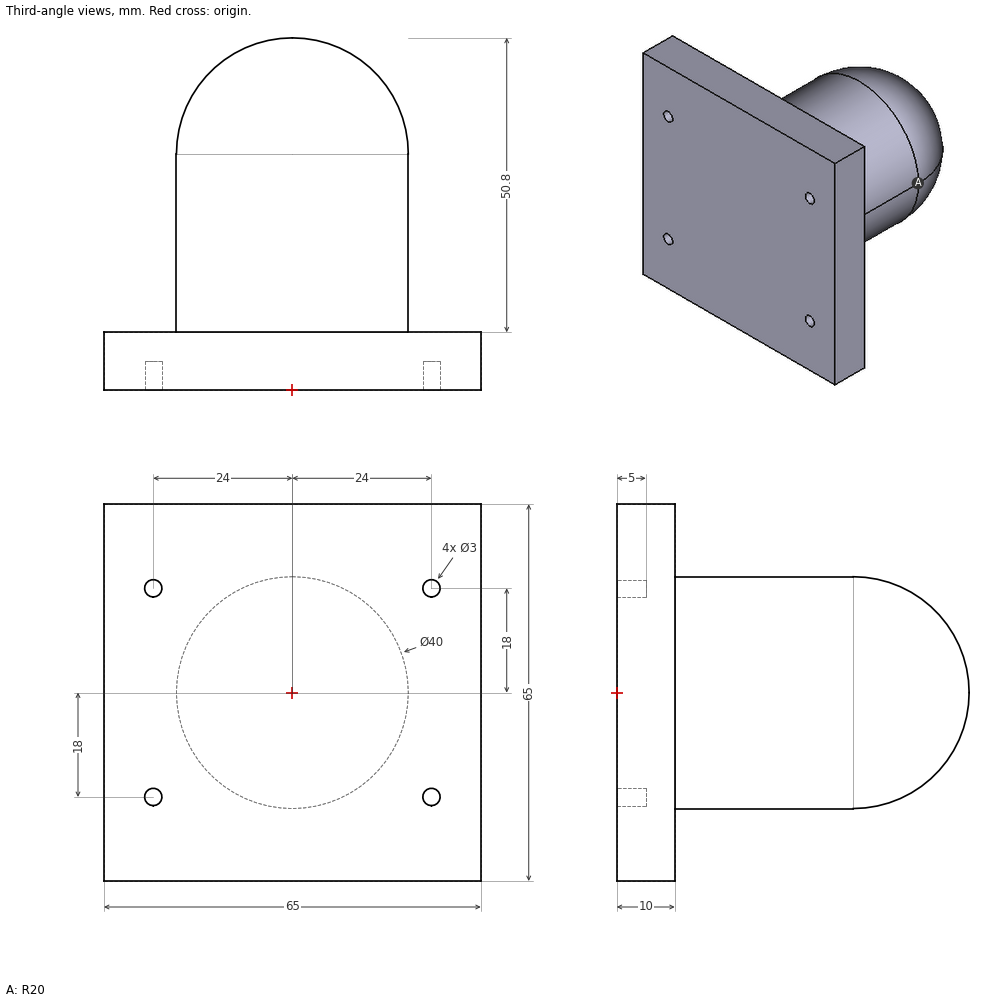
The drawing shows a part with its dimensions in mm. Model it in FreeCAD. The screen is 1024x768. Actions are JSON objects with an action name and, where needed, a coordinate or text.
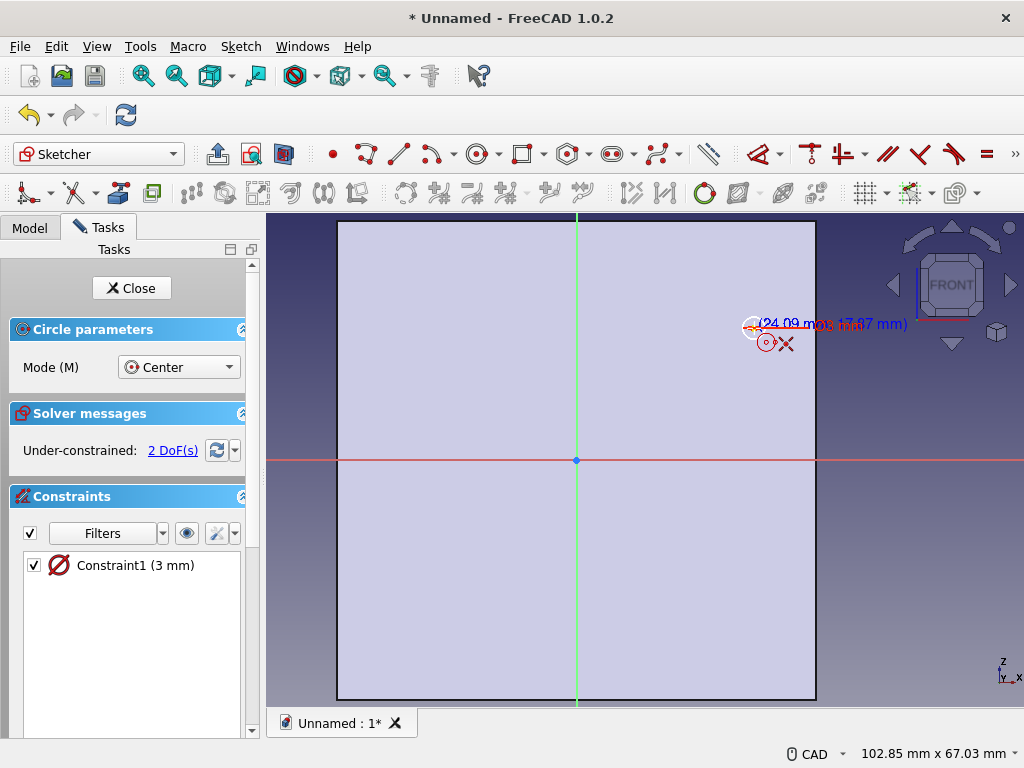
{"action": "scroll", "coordinate": [400, 328], "scroll_direction": "up", "scroll_amount": 4}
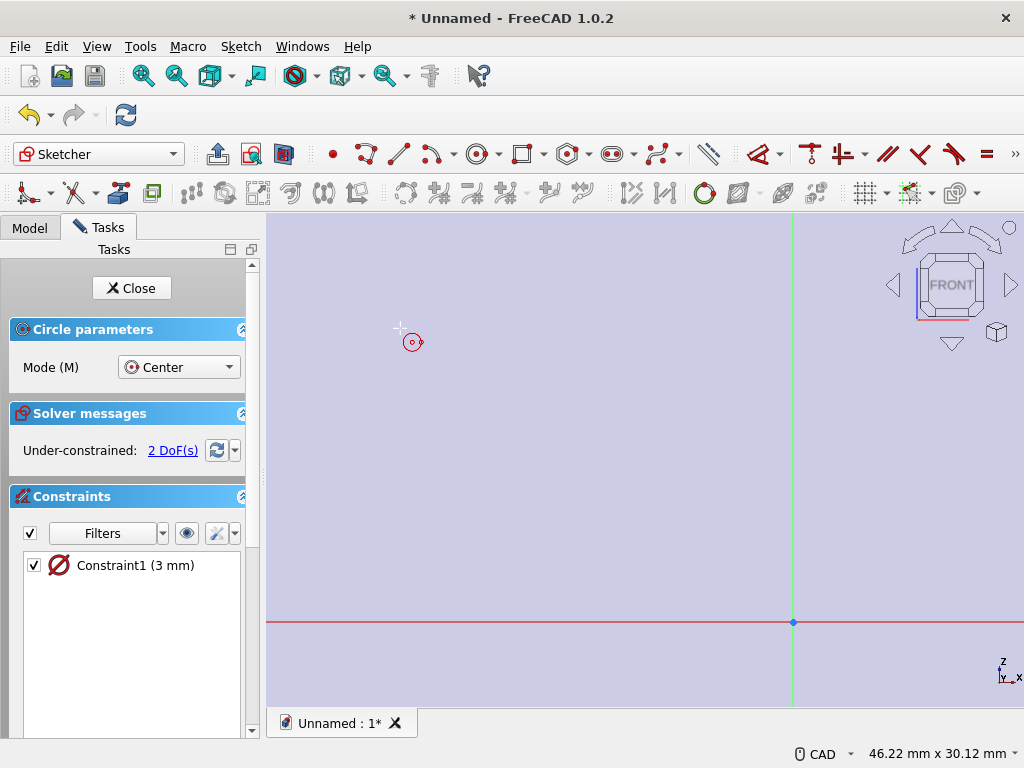
{"action": "left_click", "coordinate": [400, 327]}
{"action": "mouse_move", "coordinate": [417, 310]}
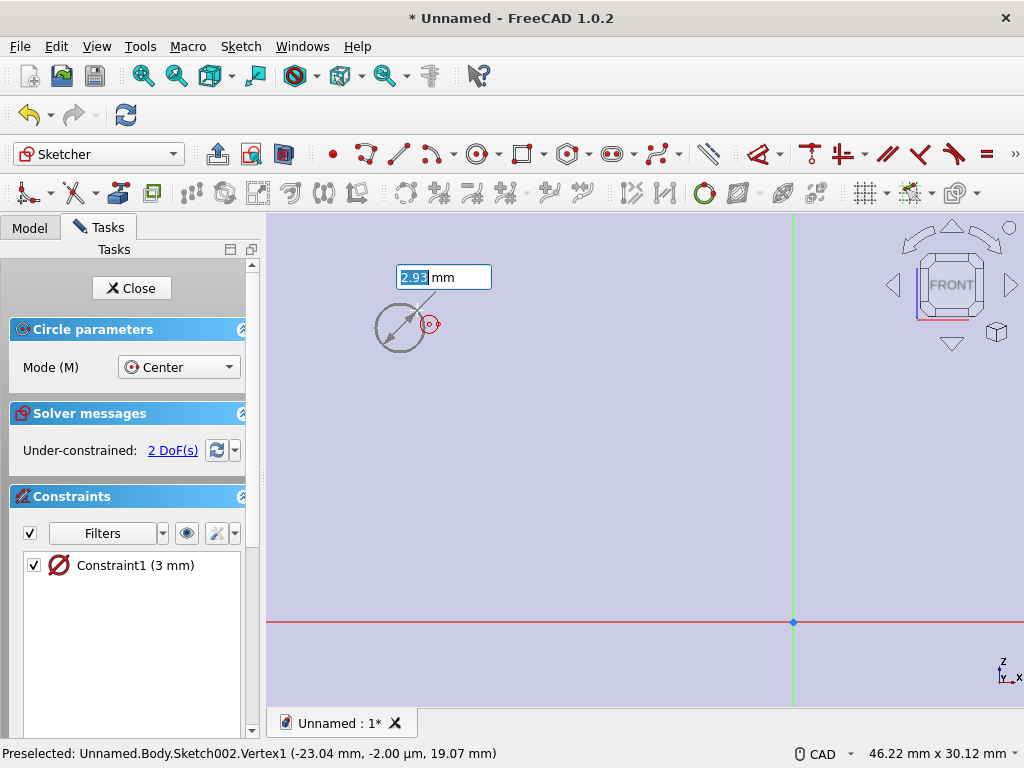
{"action": "type", "text": "3"}
{"action": "key", "text": "Return"}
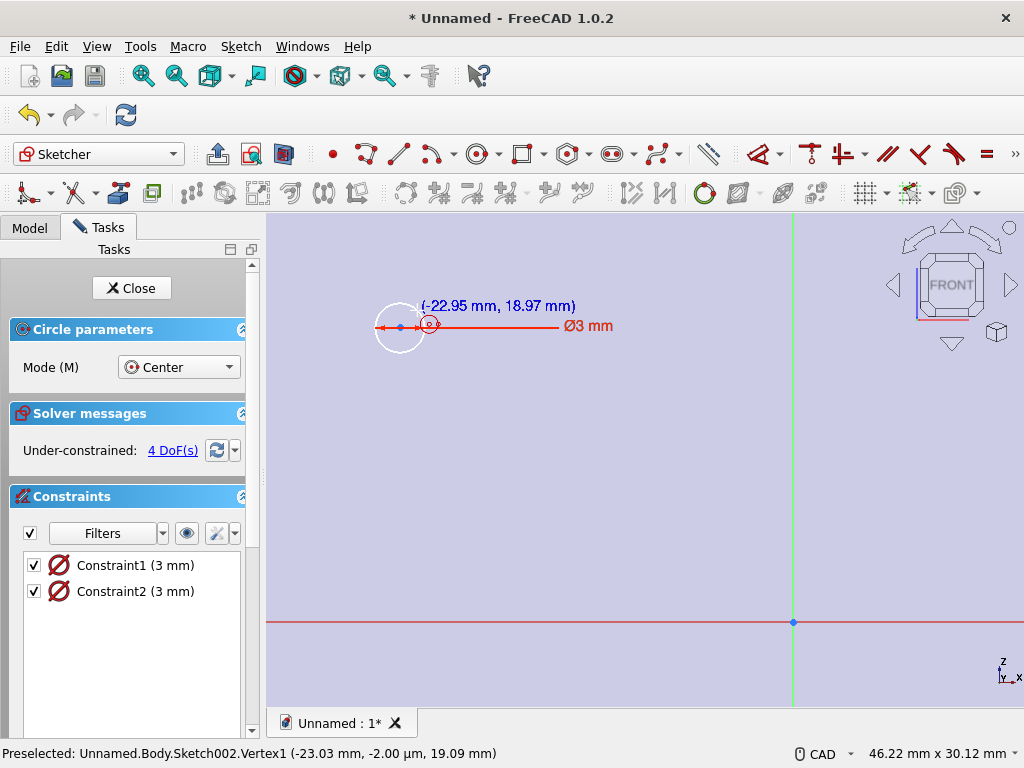
{"action": "scroll", "coordinate": [400, 328], "scroll_direction": "down", "scroll_amount": 4}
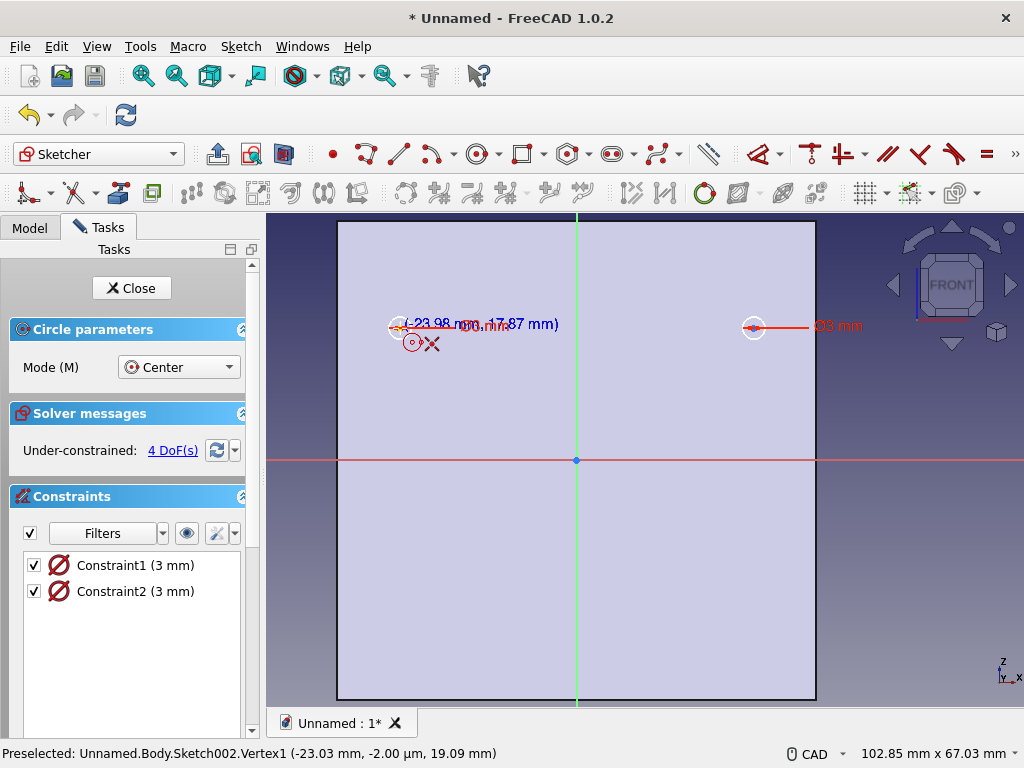
{"action": "scroll", "coordinate": [400, 593], "scroll_direction": "up", "scroll_amount": 4}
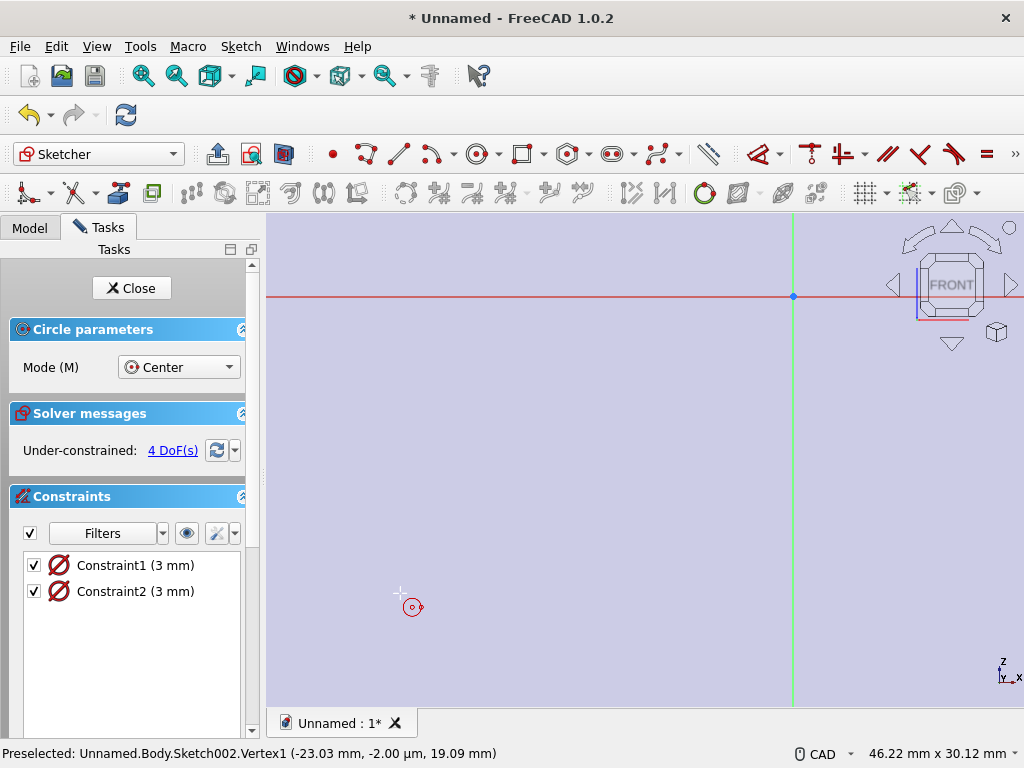
{"action": "left_click", "coordinate": [400, 592]}
{"action": "mouse_move", "coordinate": [417, 575]}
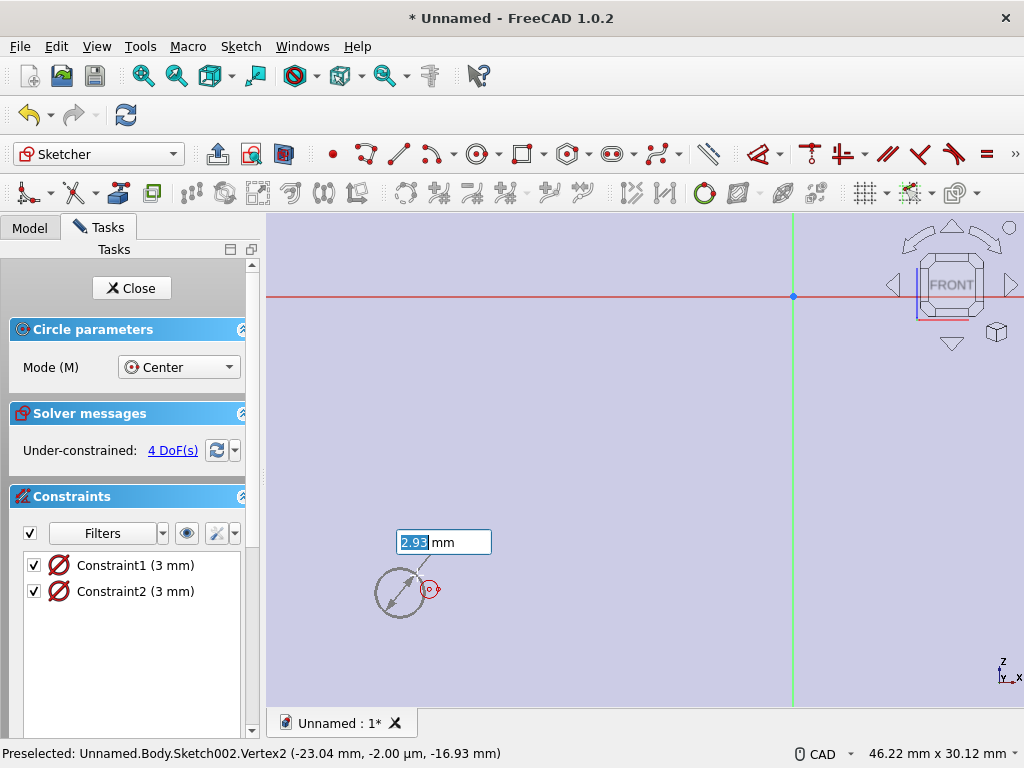
{"action": "type", "text": "3"}
{"action": "key", "text": "Return"}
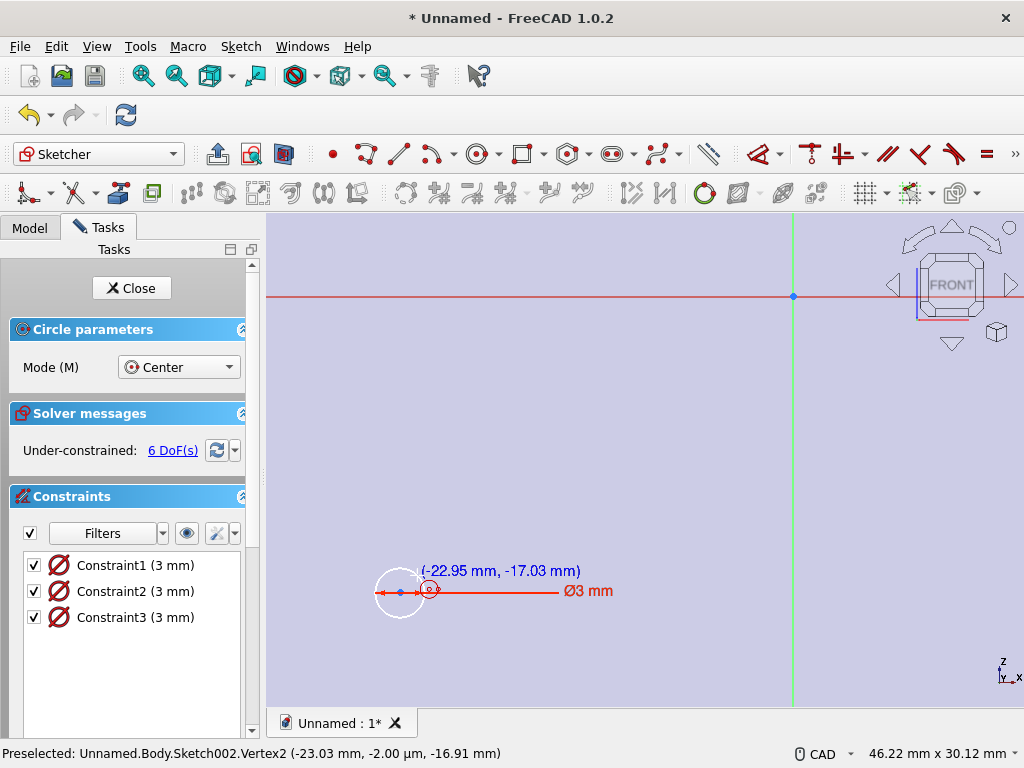
{"action": "scroll", "coordinate": [400, 593], "scroll_direction": "down", "scroll_amount": 4}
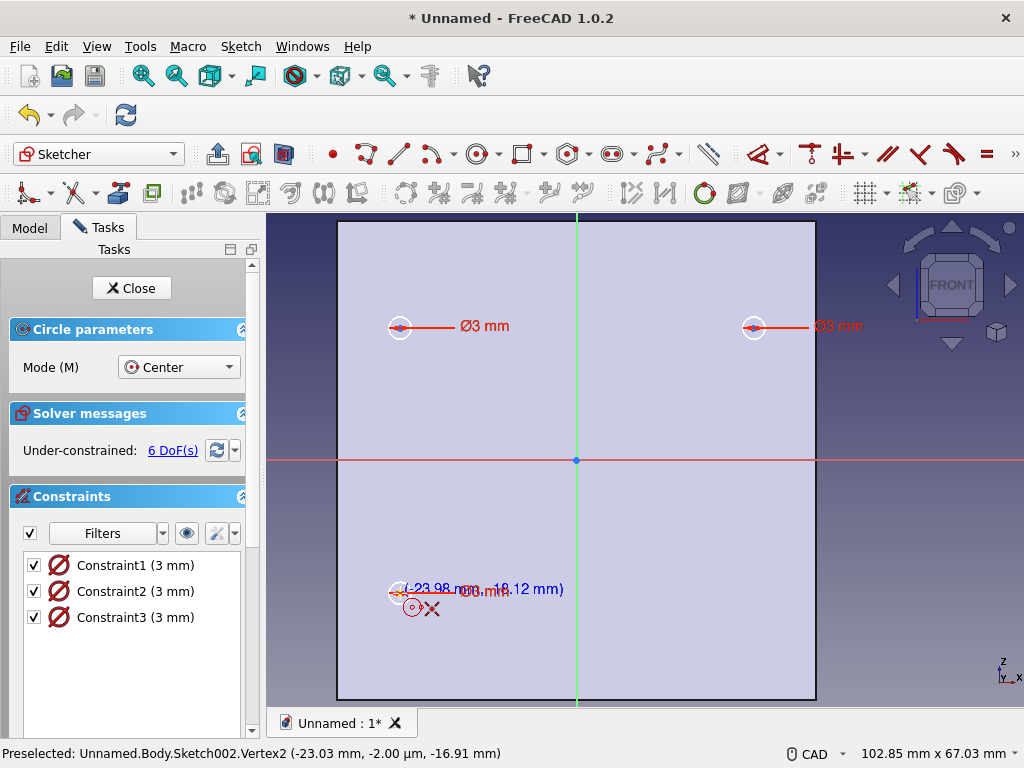
{"action": "scroll", "coordinate": [754, 593], "scroll_direction": "up", "scroll_amount": 4}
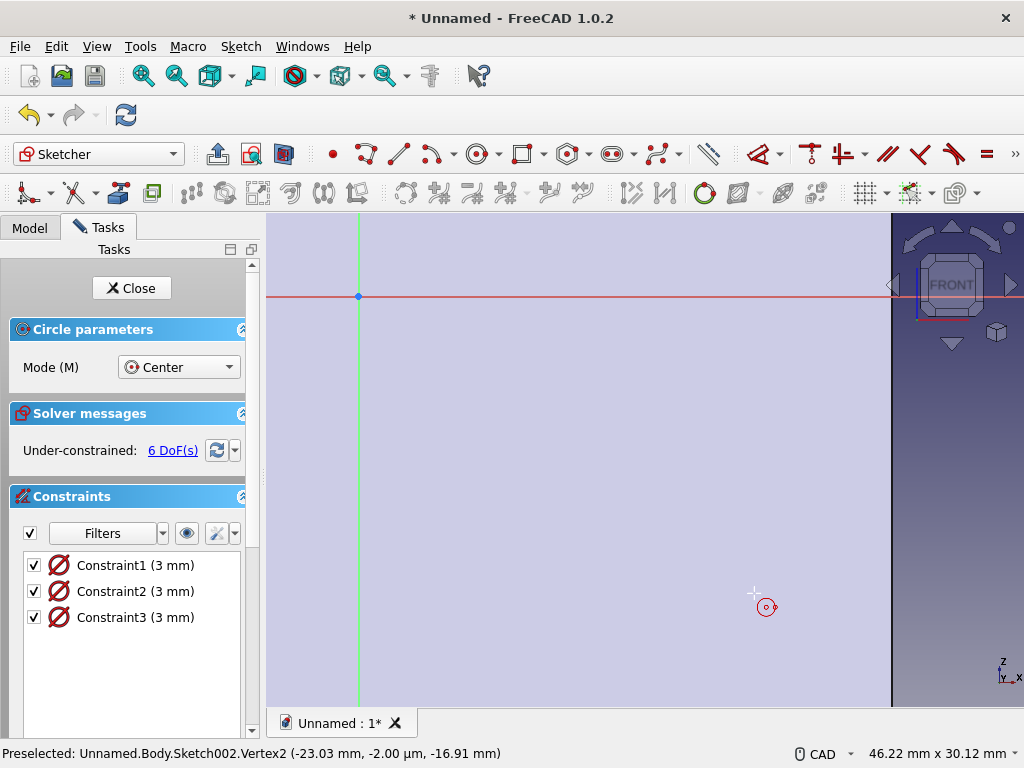
{"action": "left_click", "coordinate": [753, 592]}
{"action": "mouse_move", "coordinate": [770, 575]}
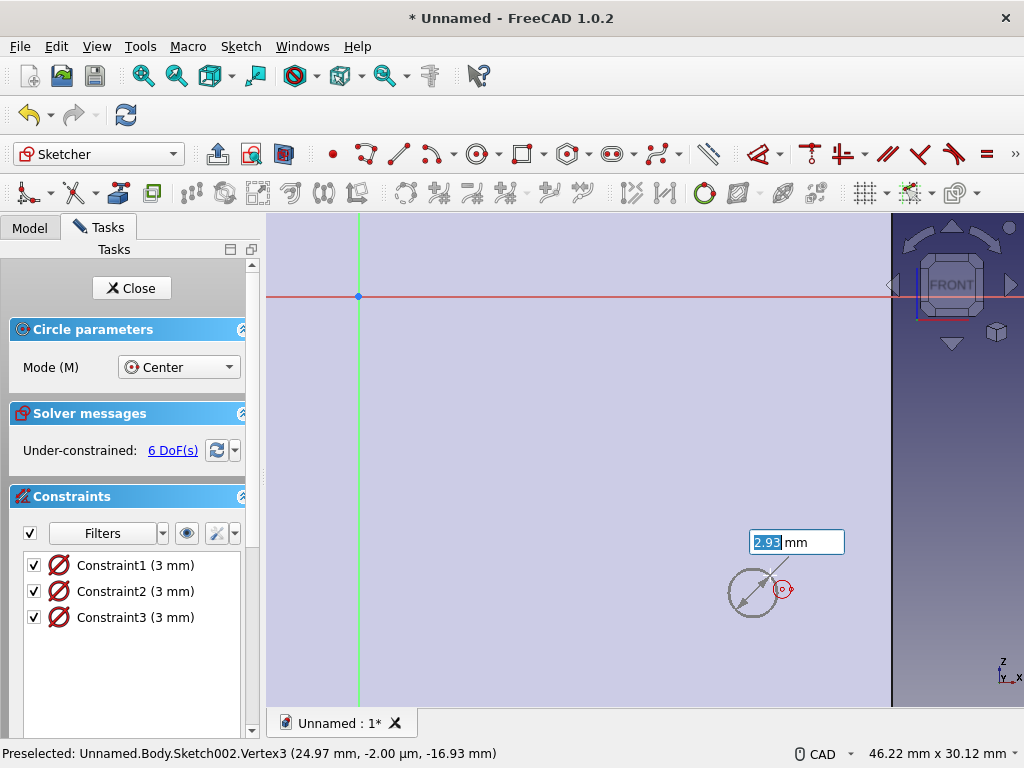
{"action": "type", "text": "3"}
{"action": "key", "text": "Return"}
{"action": "key", "text": "Escape"}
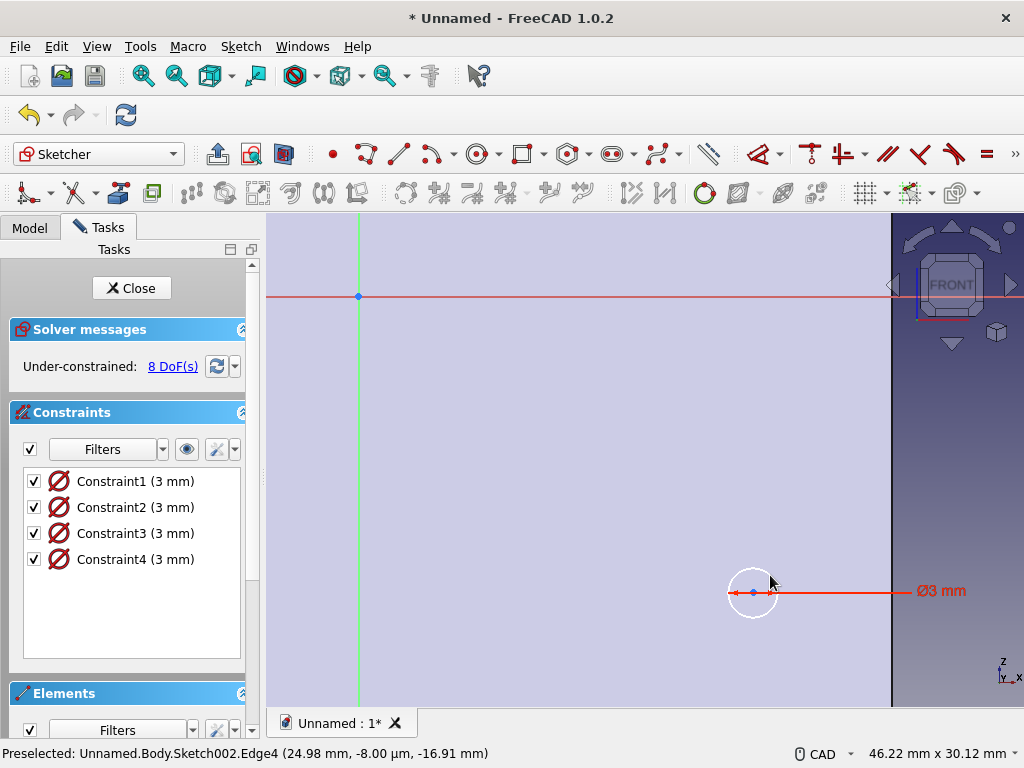
{"action": "scroll", "coordinate": [754, 593], "scroll_direction": "down", "scroll_amount": 4}